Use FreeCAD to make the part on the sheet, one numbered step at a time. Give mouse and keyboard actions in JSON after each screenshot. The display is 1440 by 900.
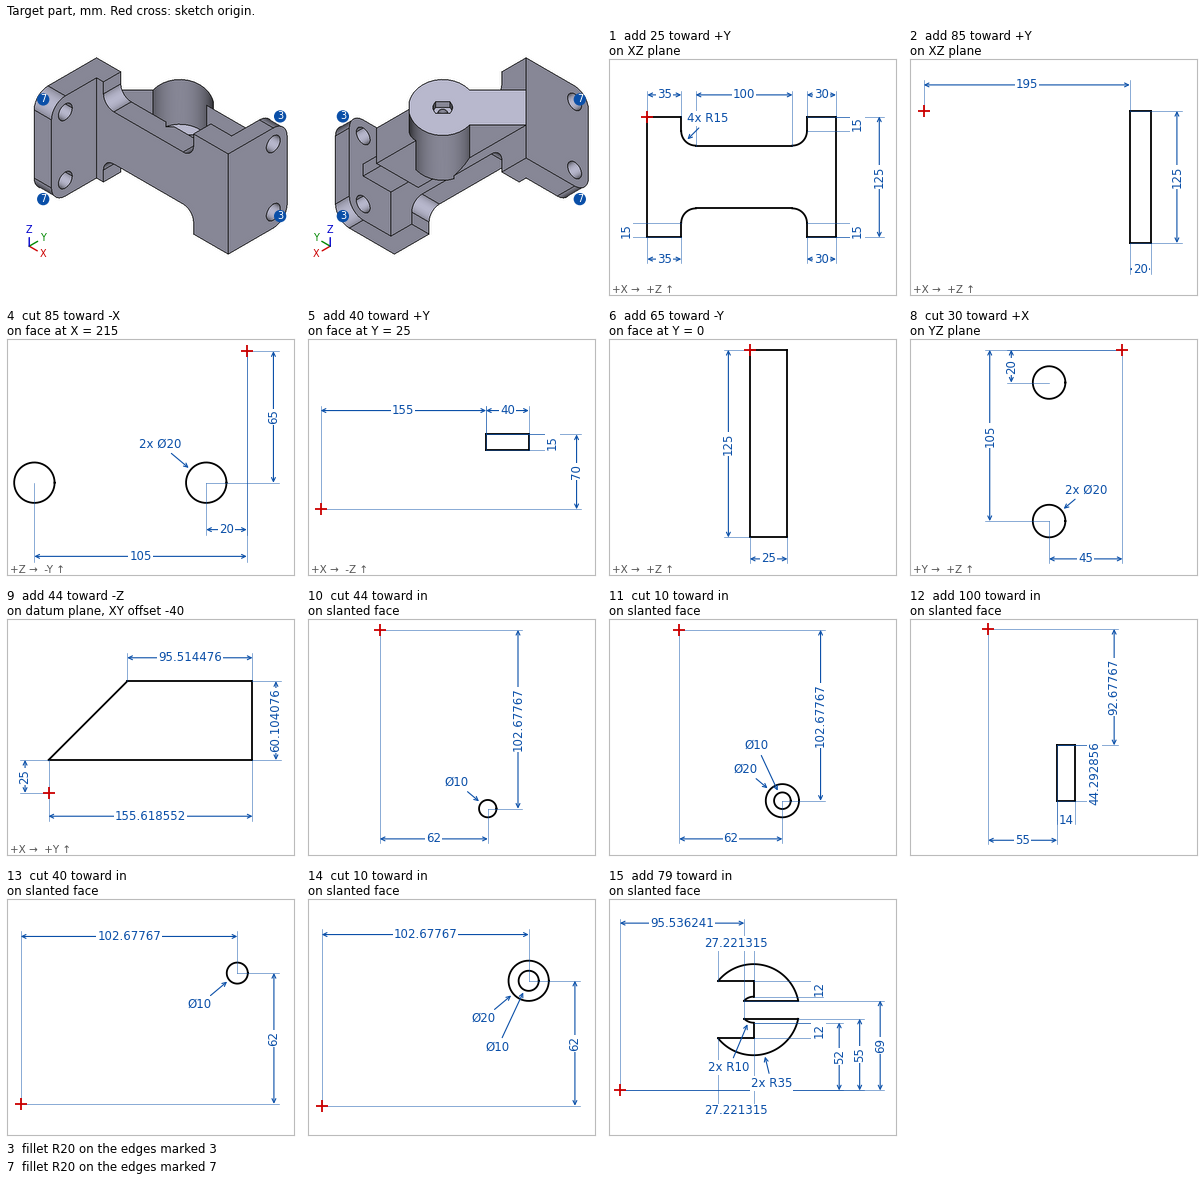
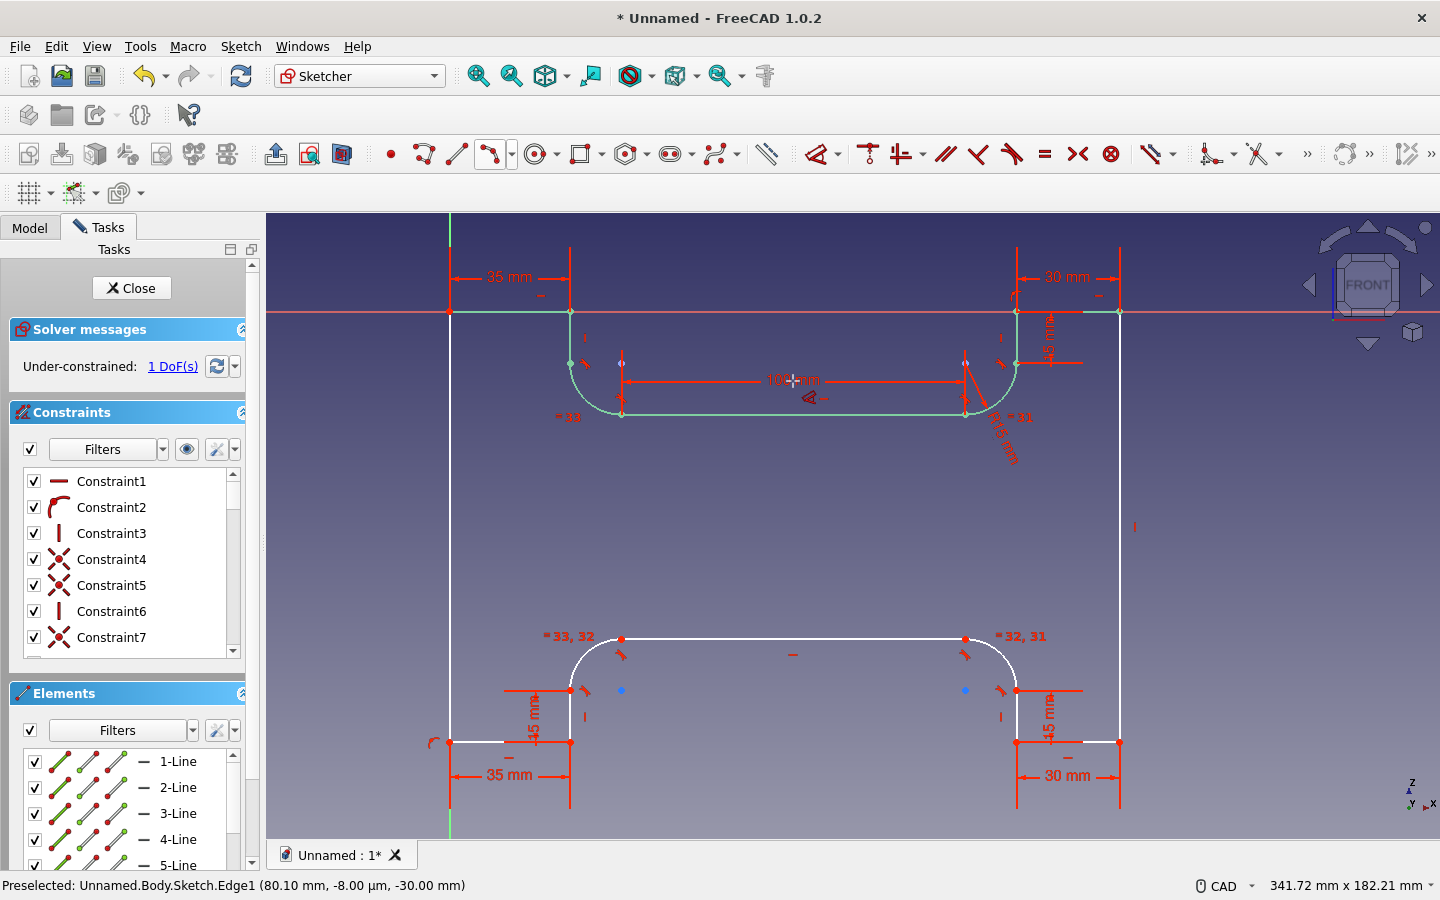
{"action": "left_click", "coordinate": [1120, 441]}
{"action": "left_click", "coordinate": [1154, 527]}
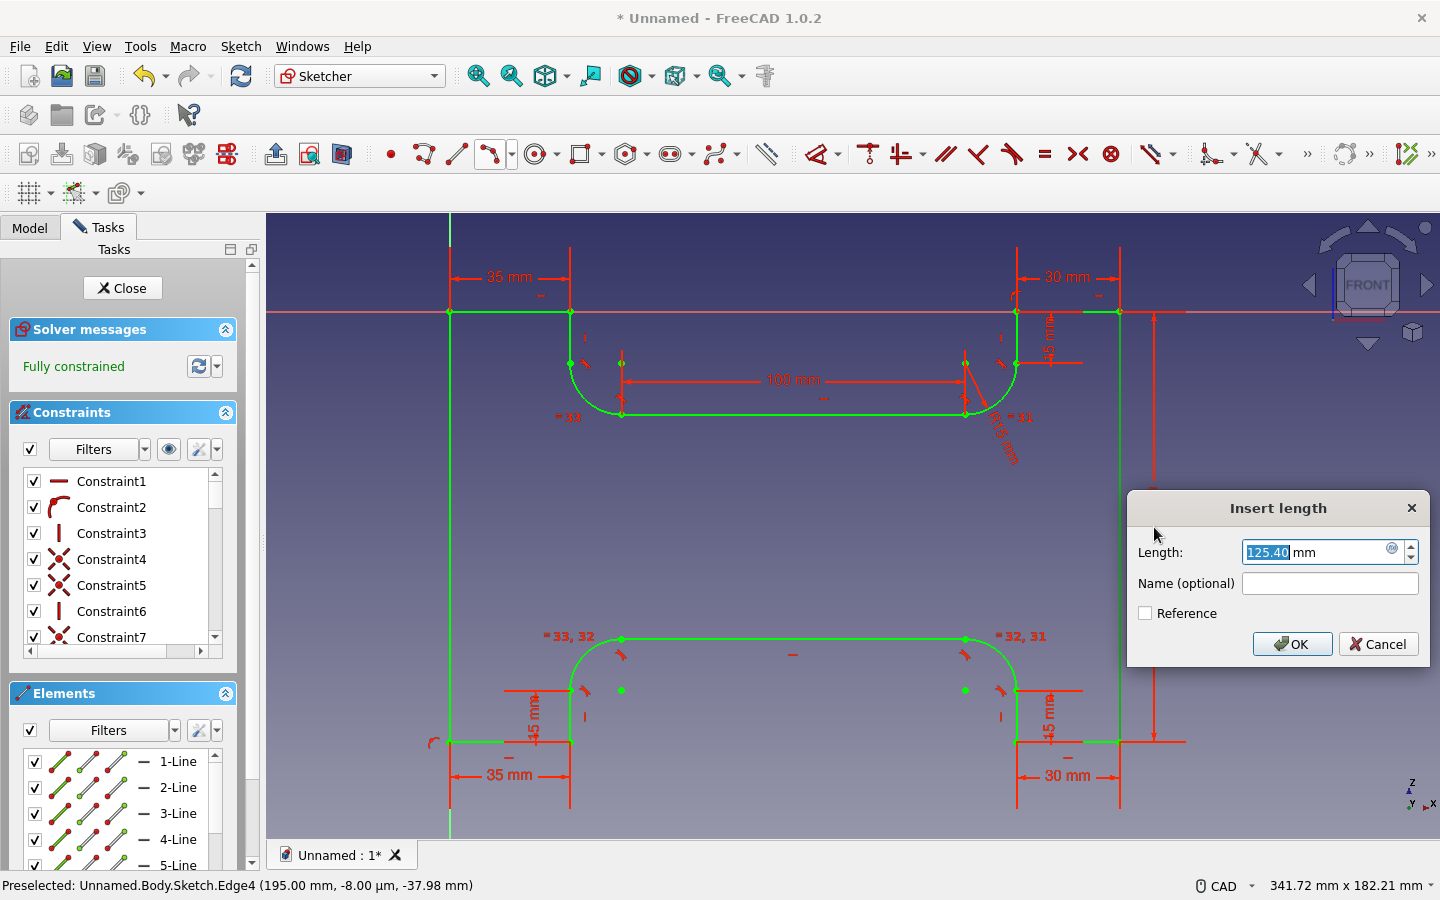
{"action": "type", "text": "125"}
{"action": "key", "text": "Return"}
{"action": "key", "text": "Escape"}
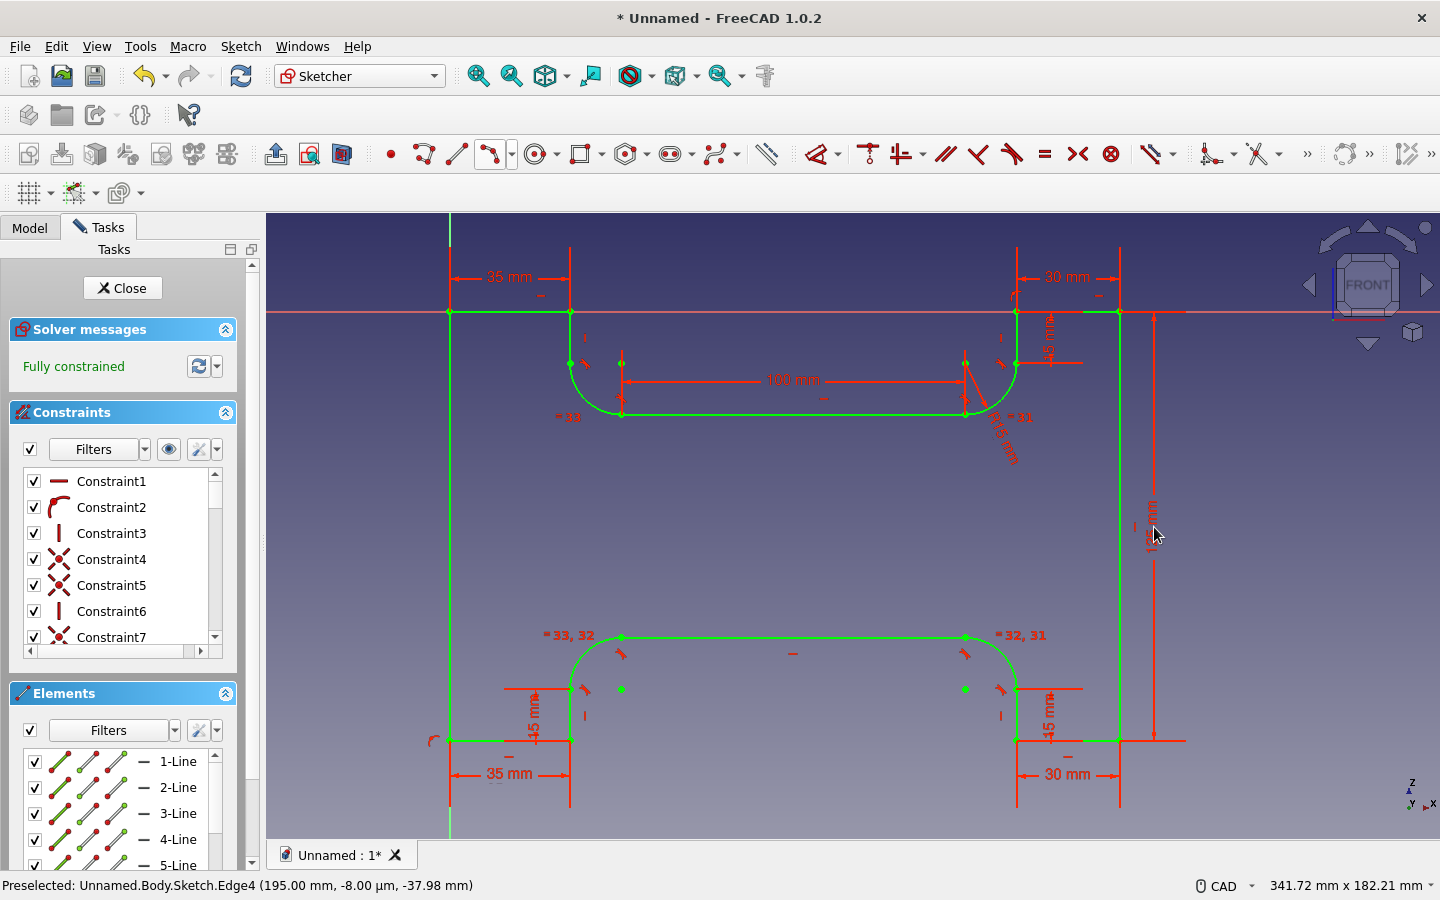
{"action": "left_click", "coordinate": [123, 288]}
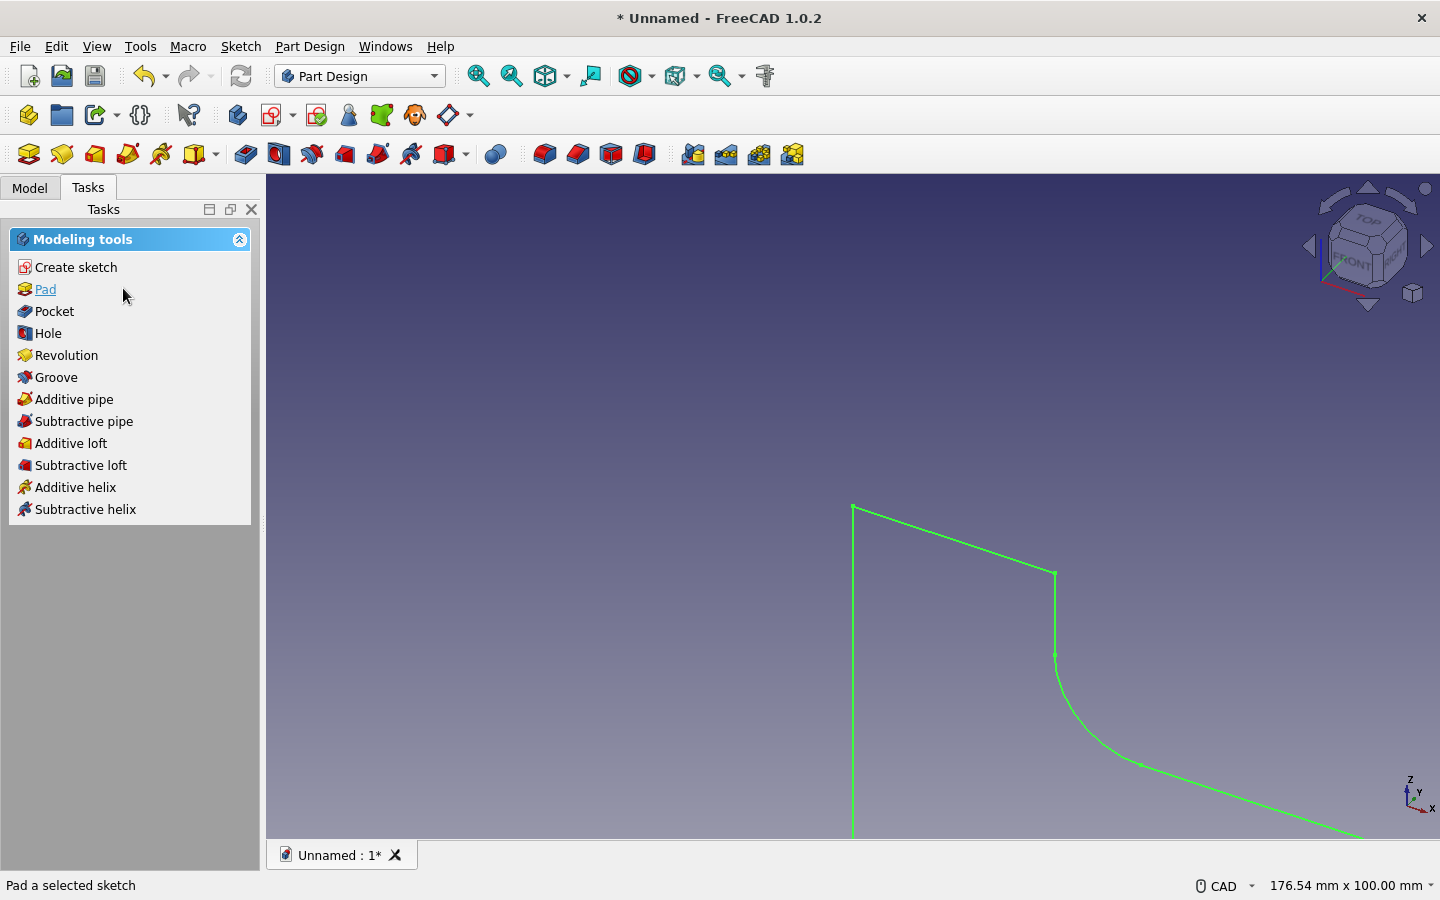
{"action": "left_click", "coordinate": [29, 154]}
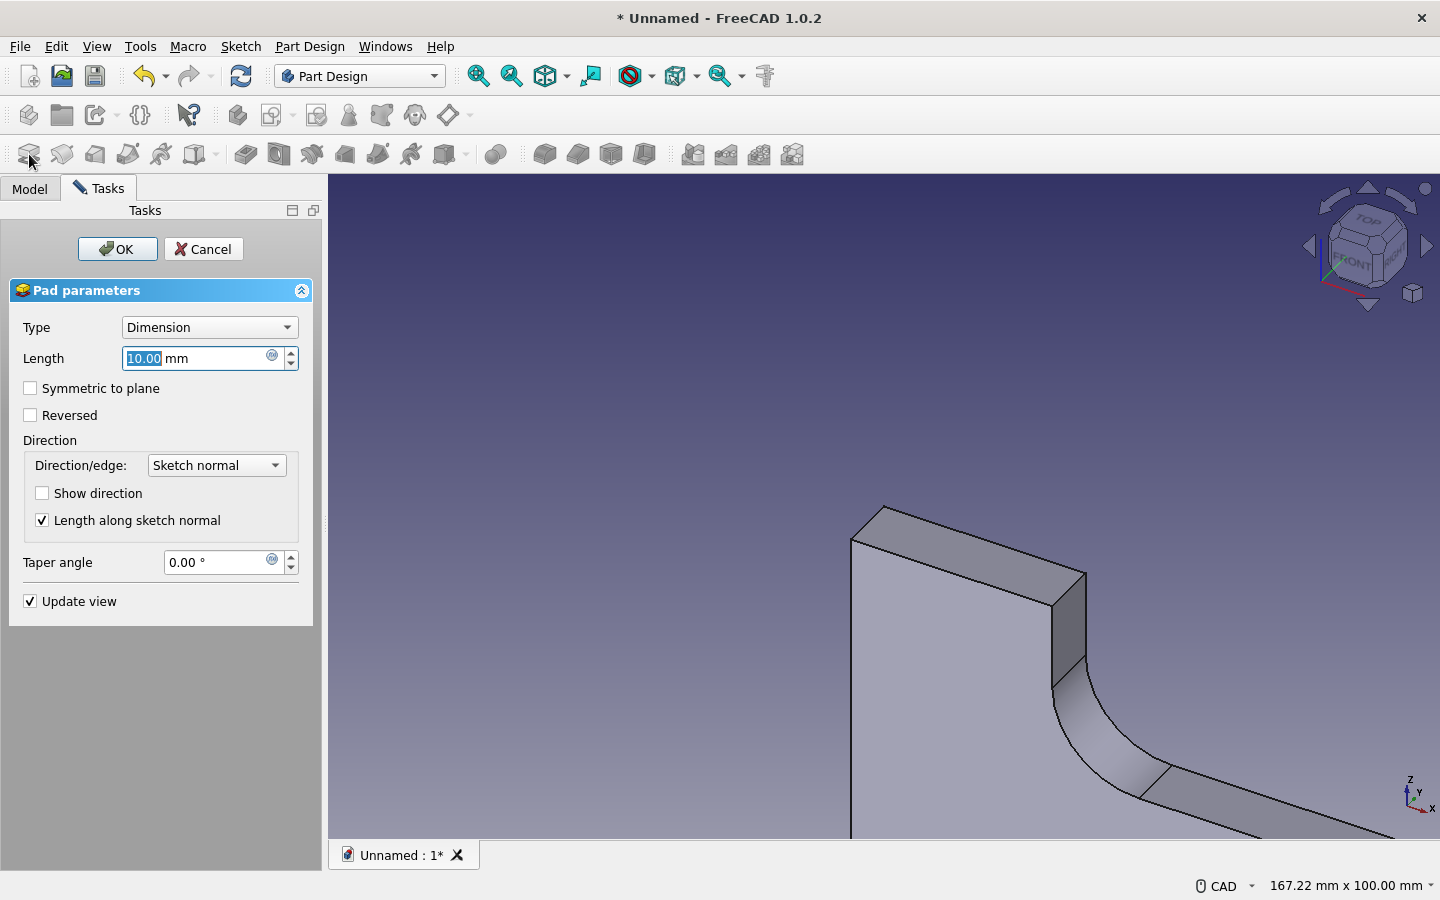
{"action": "type", "text": "25"}
{"action": "key", "text": "Tab"}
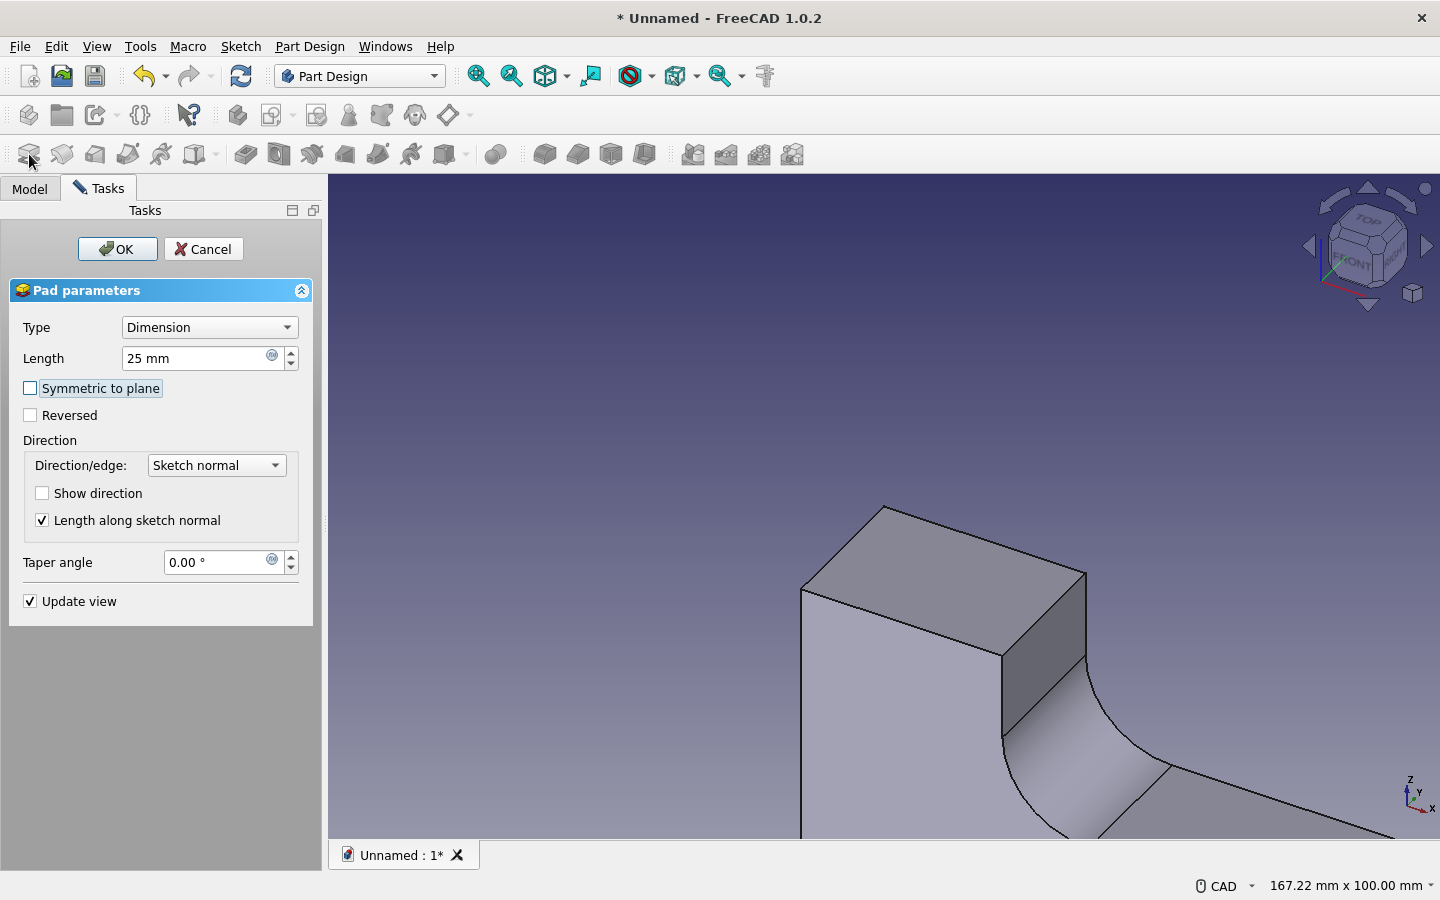
{"action": "left_click", "coordinate": [31, 415]}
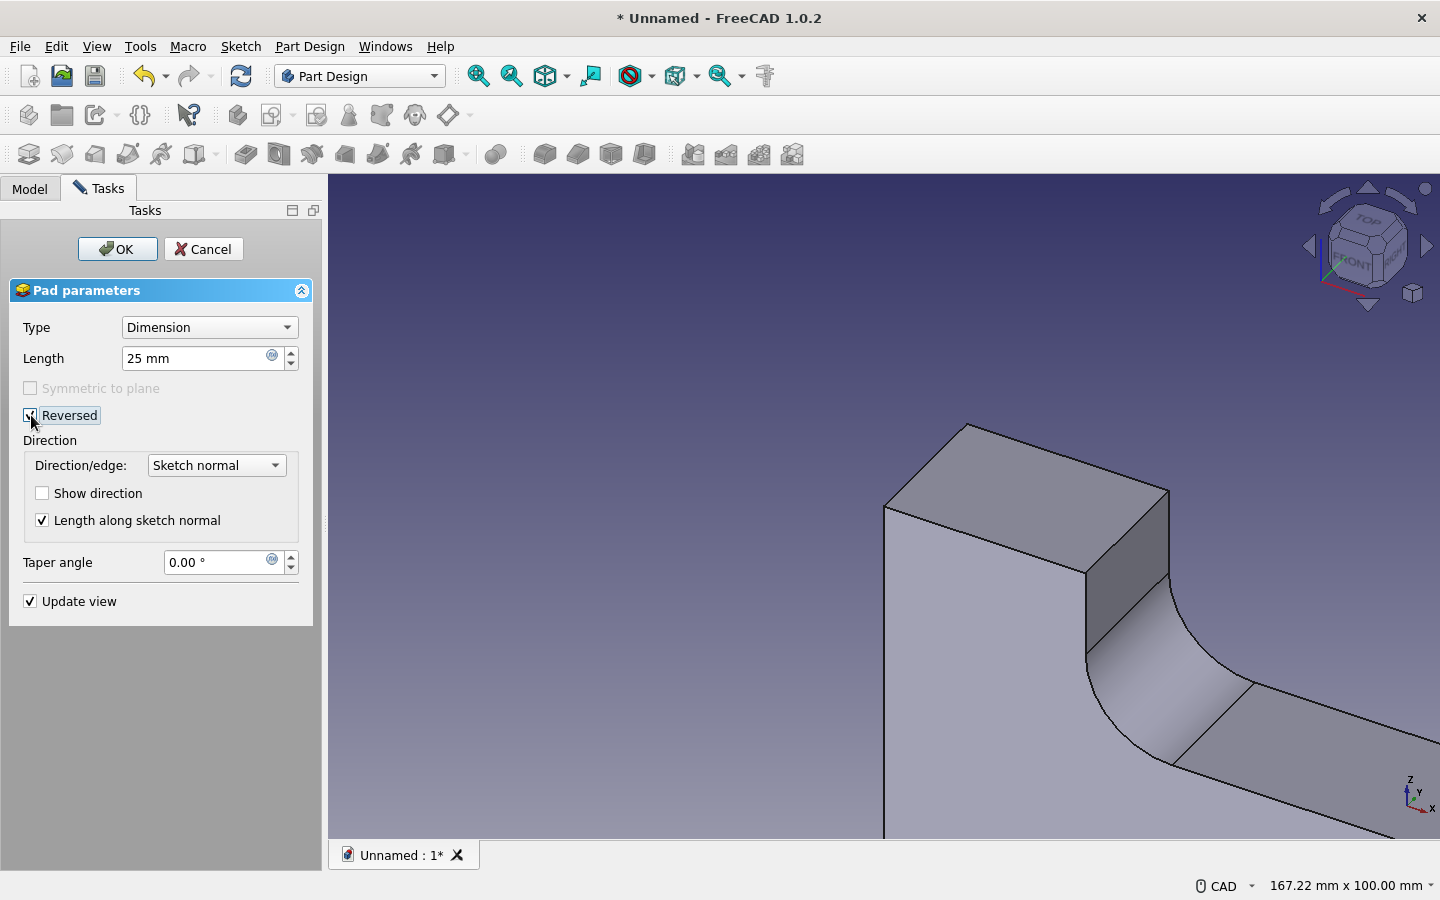
{"action": "left_click", "coordinate": [118, 249]}